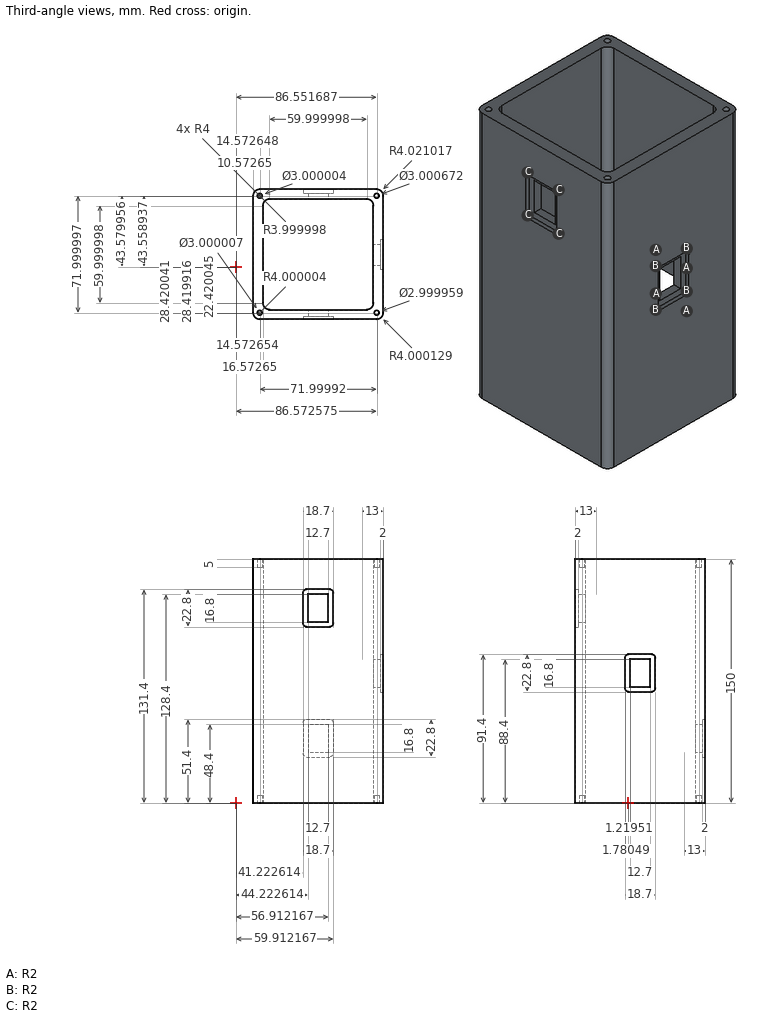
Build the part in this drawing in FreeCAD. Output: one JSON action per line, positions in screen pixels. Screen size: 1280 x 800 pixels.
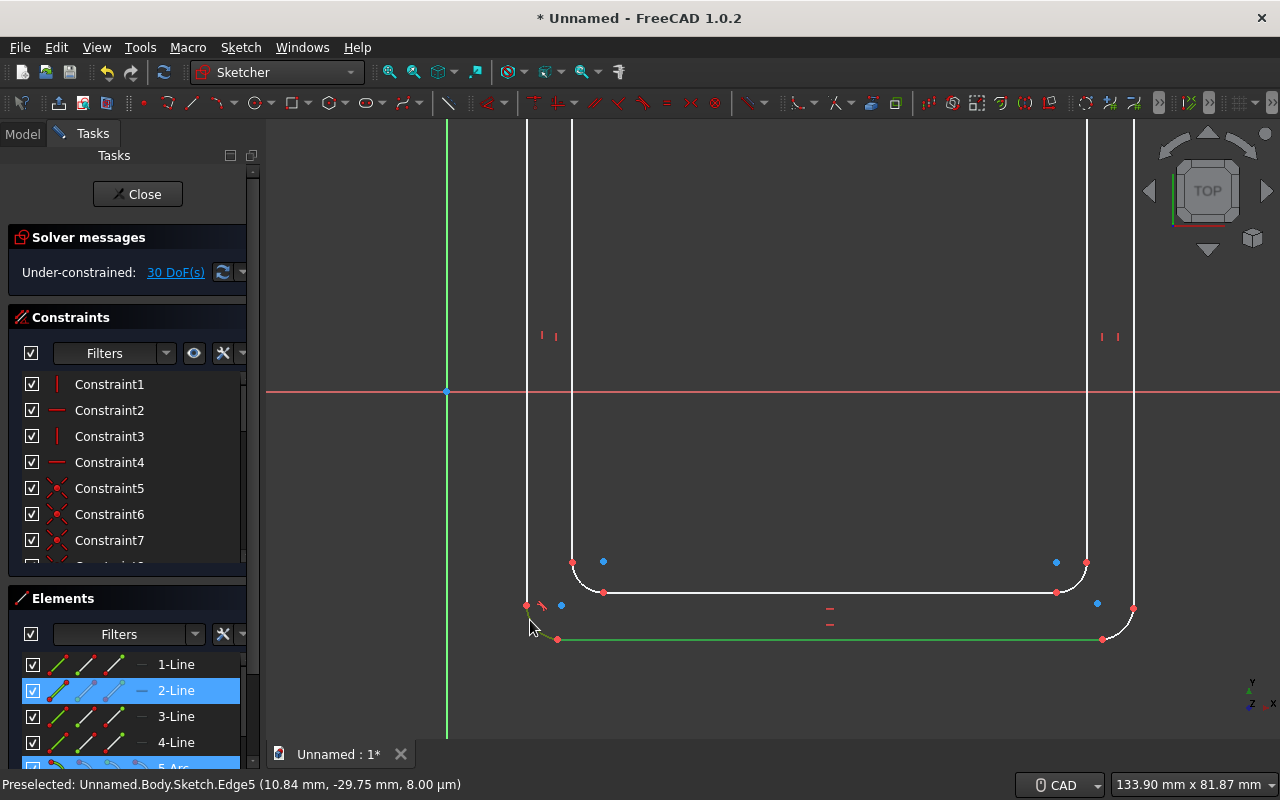
{"action": "left_click", "coordinate": [644, 104]}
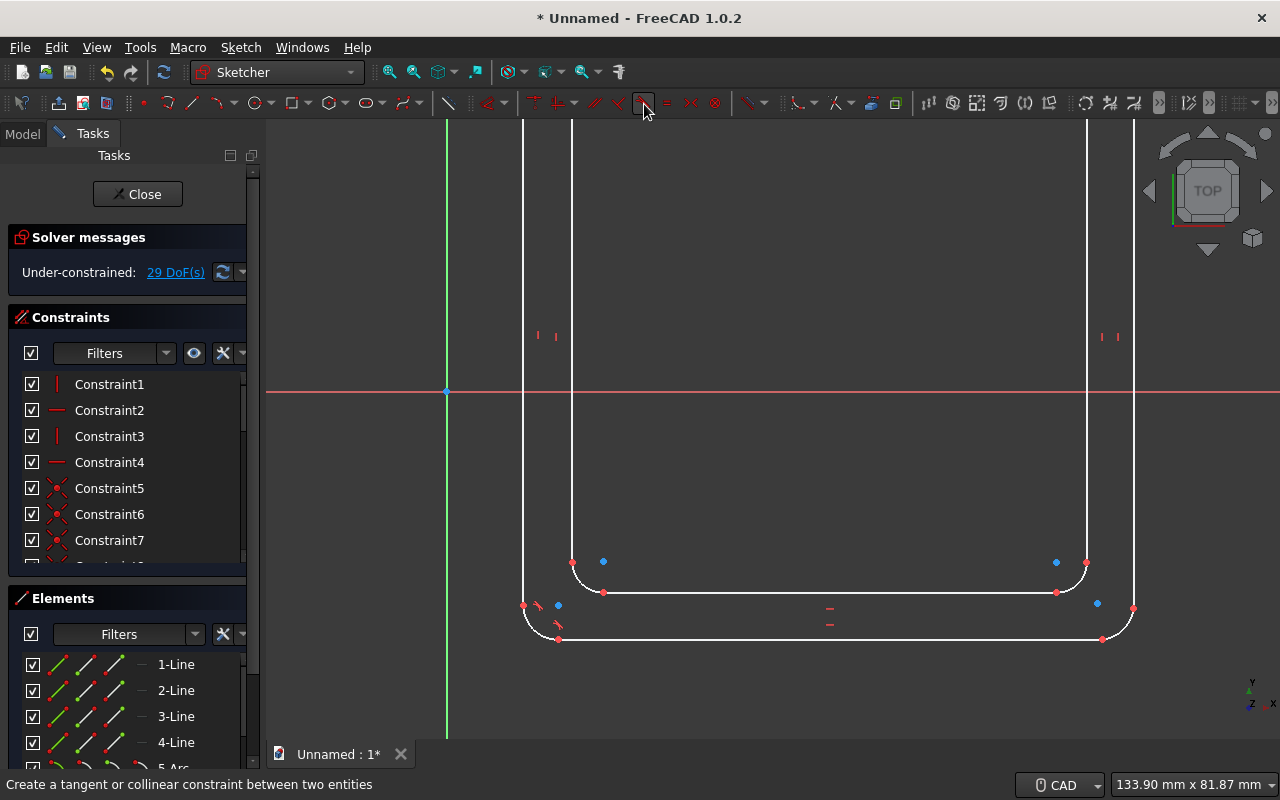
{"action": "left_click", "coordinate": [721, 640]}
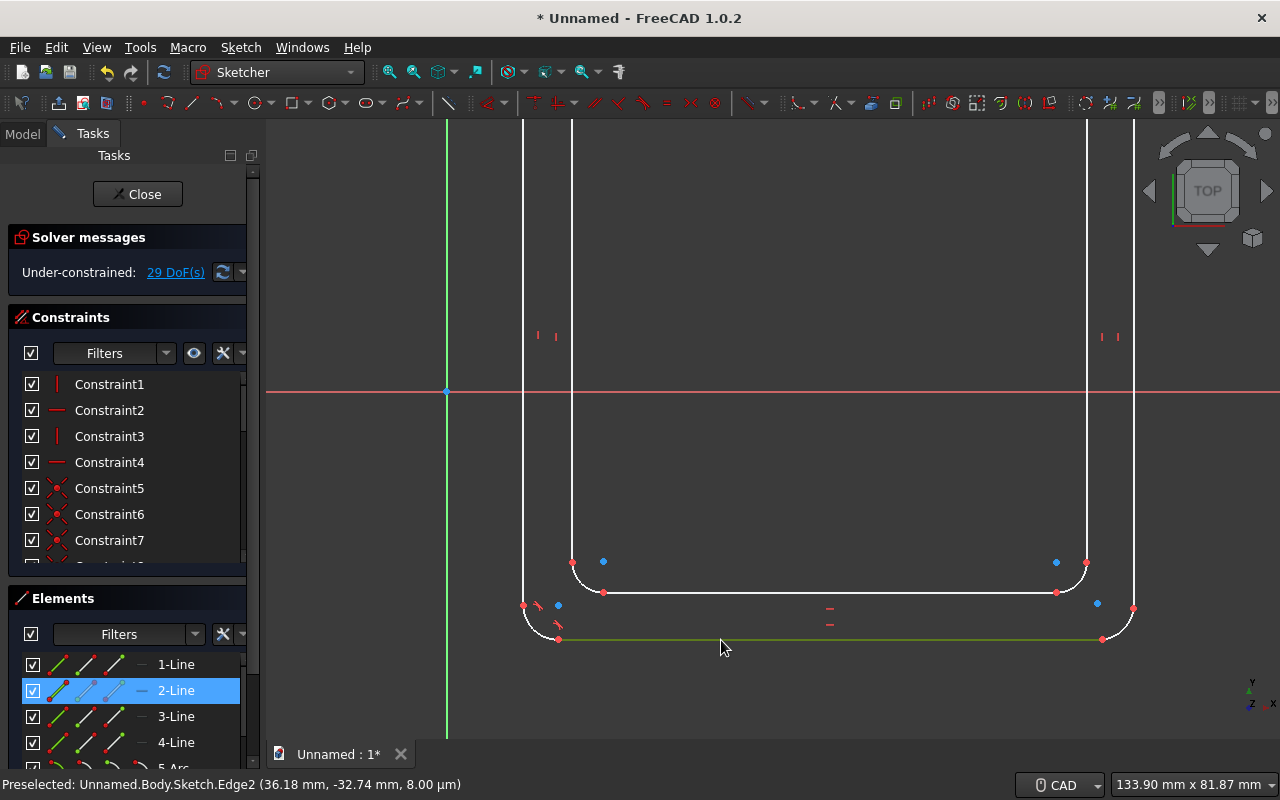
{"action": "scroll", "coordinate": [1112, 637], "scroll_direction": "up", "scroll_amount": 2}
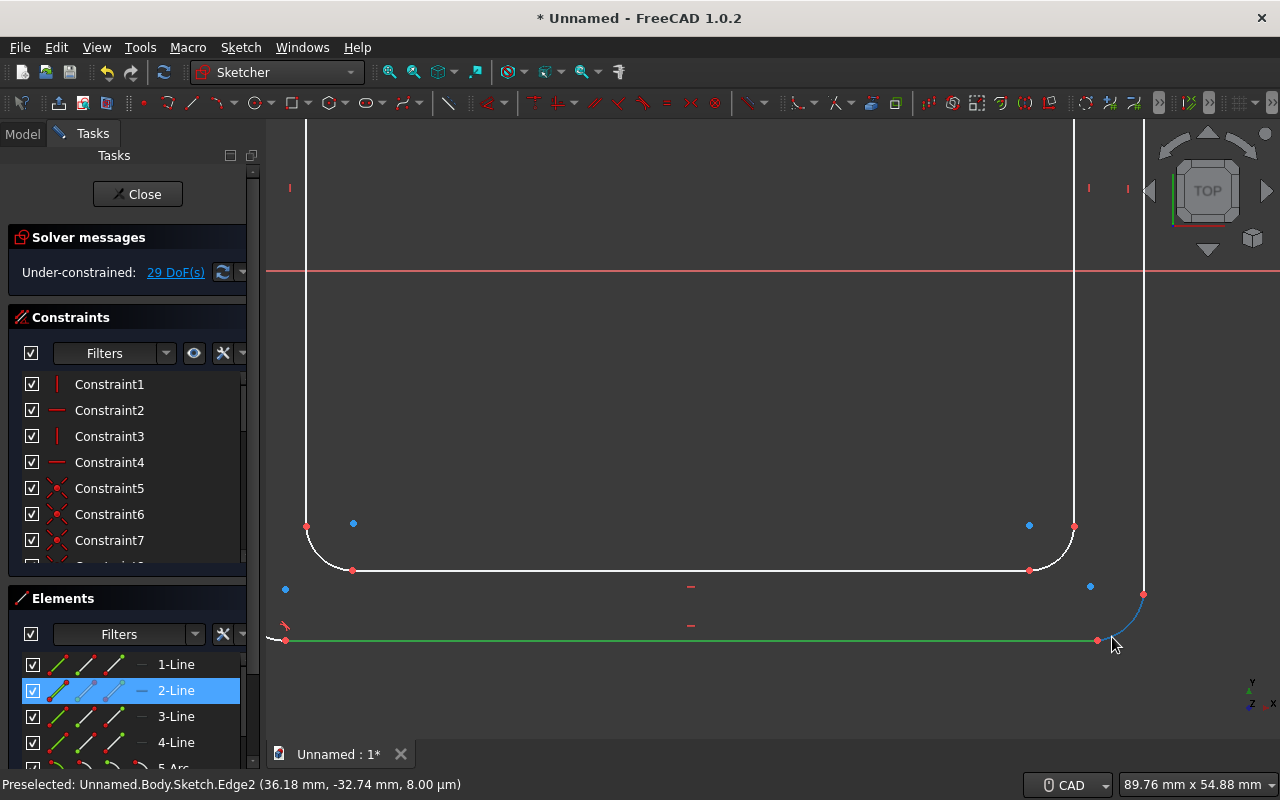
{"action": "left_click", "coordinate": [1111, 637]}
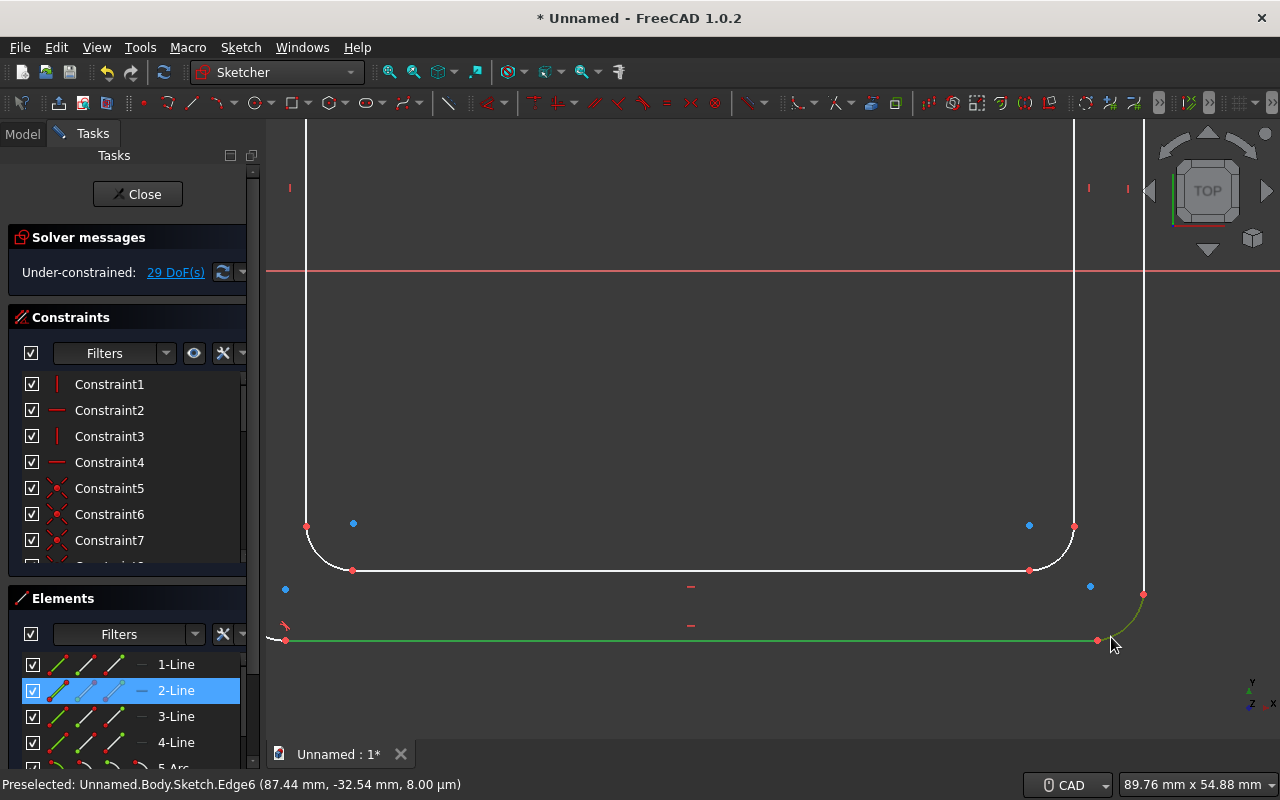
{"action": "left_click", "coordinate": [644, 104]}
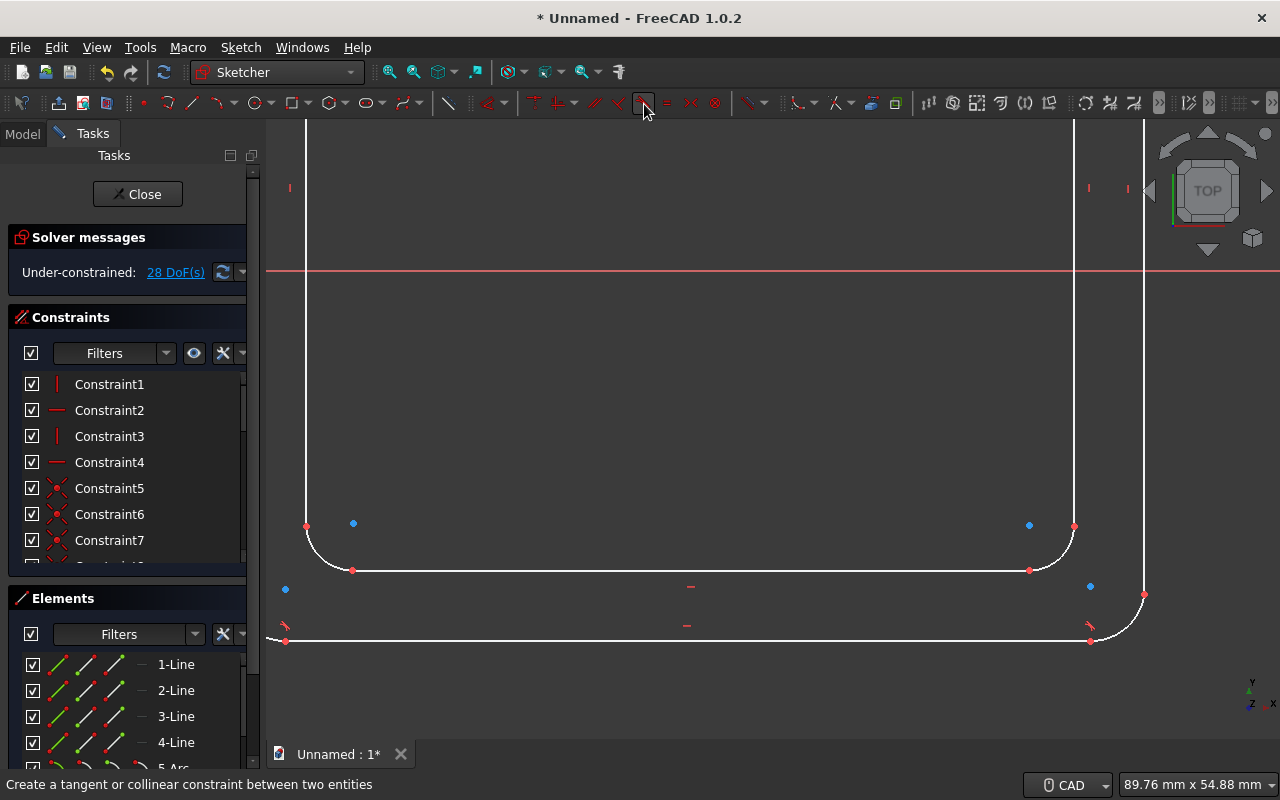
{"action": "scroll", "coordinate": [764, 628], "scroll_direction": "down", "scroll_amount": 4}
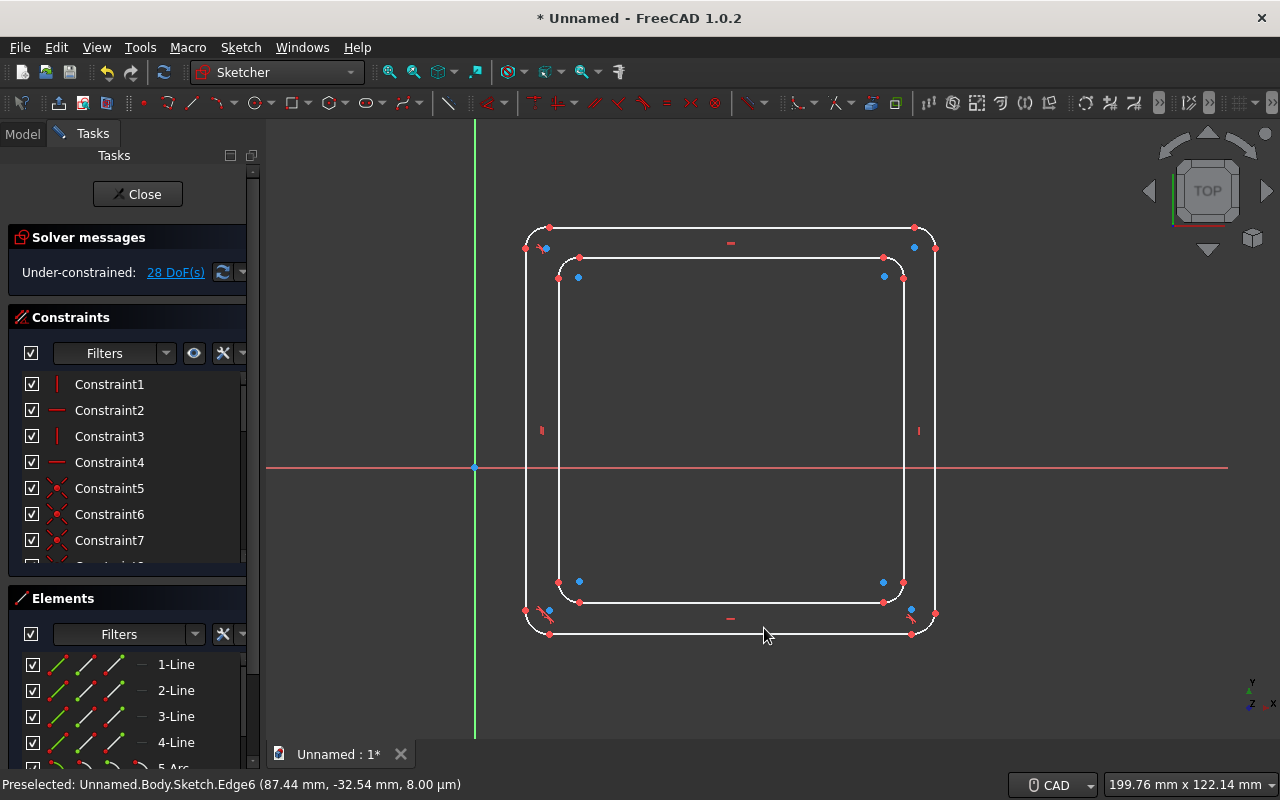
{"action": "left_click", "coordinate": [935, 504]}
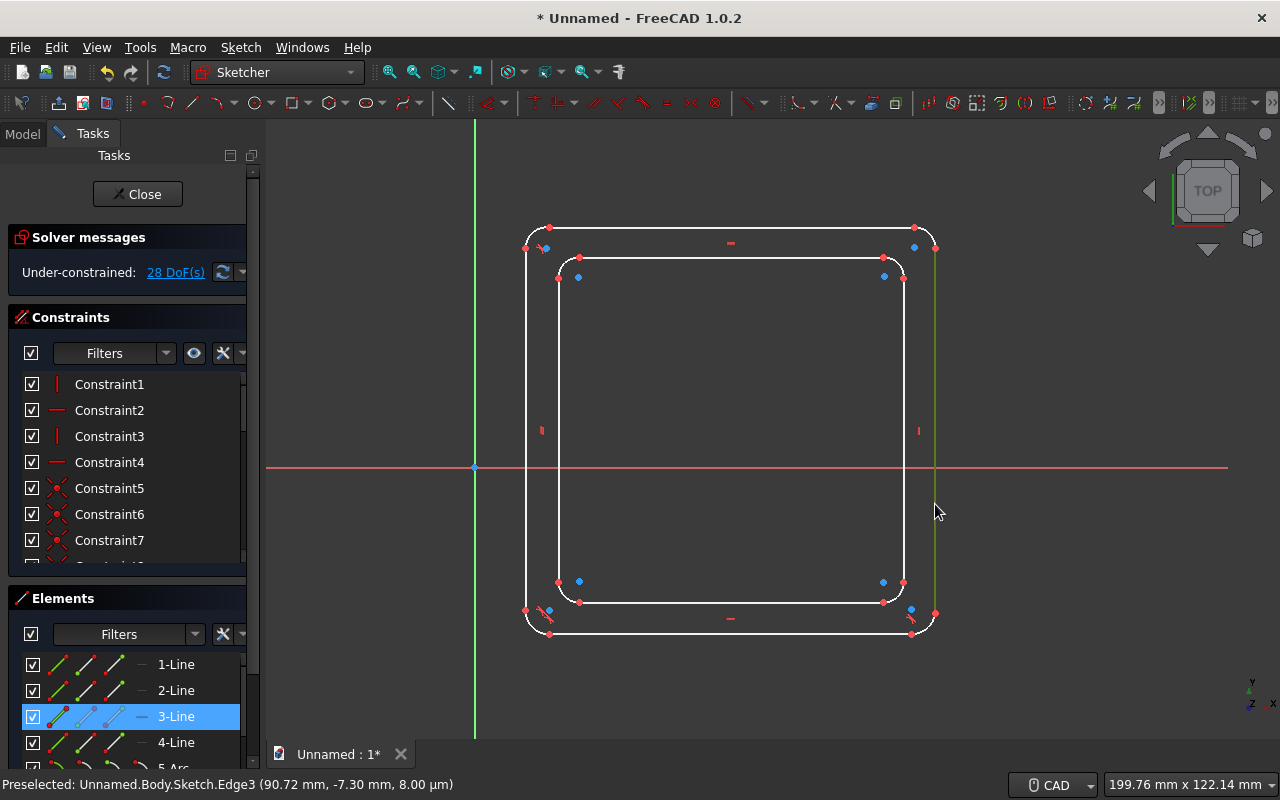
{"action": "scroll", "coordinate": [921, 632], "scroll_direction": "up", "scroll_amount": 2}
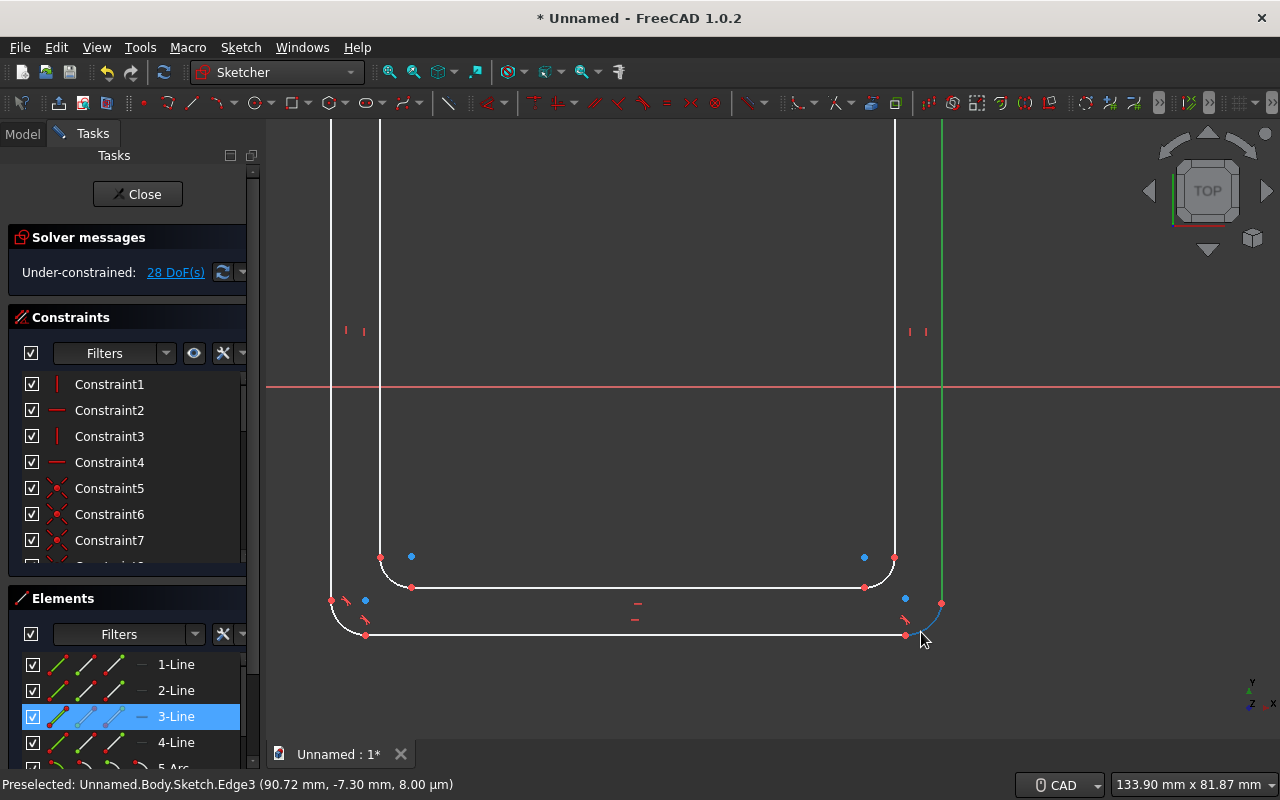
{"action": "left_click", "coordinate": [921, 632]}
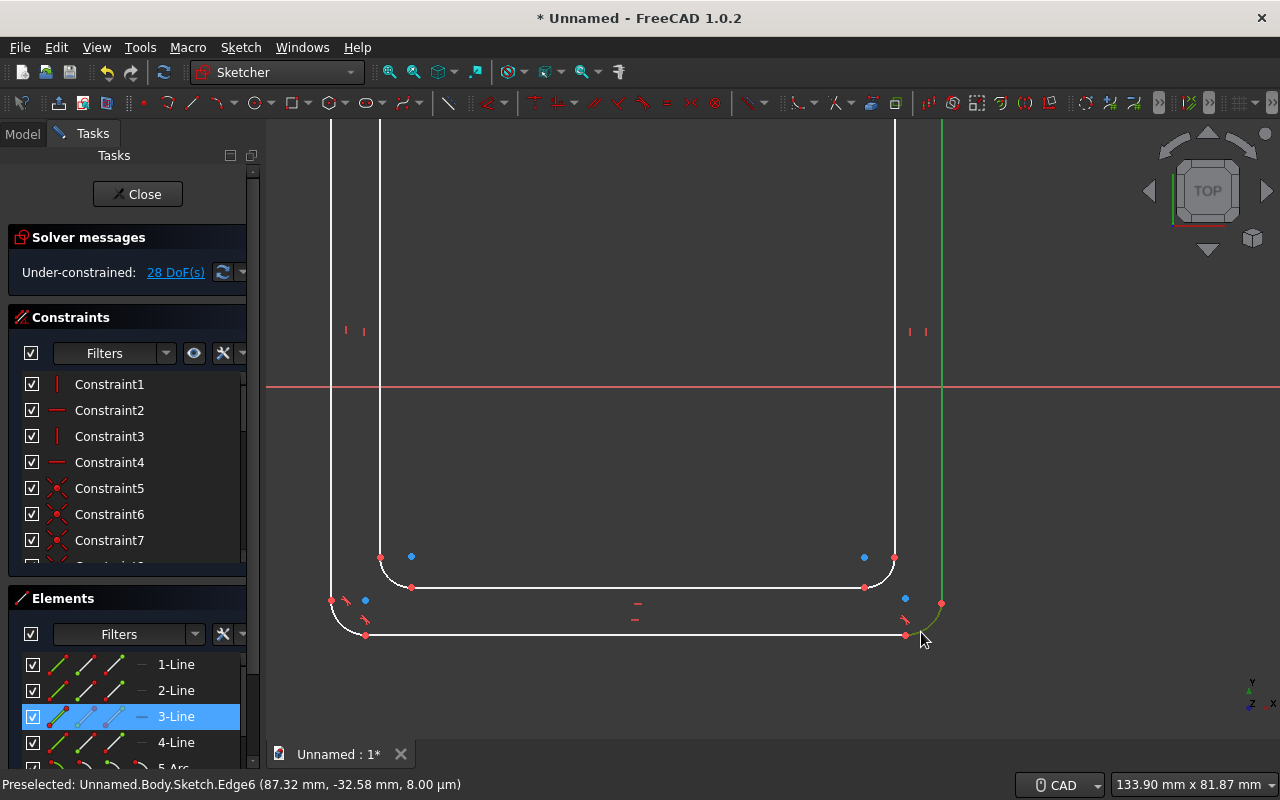
{"action": "left_click", "coordinate": [644, 104]}